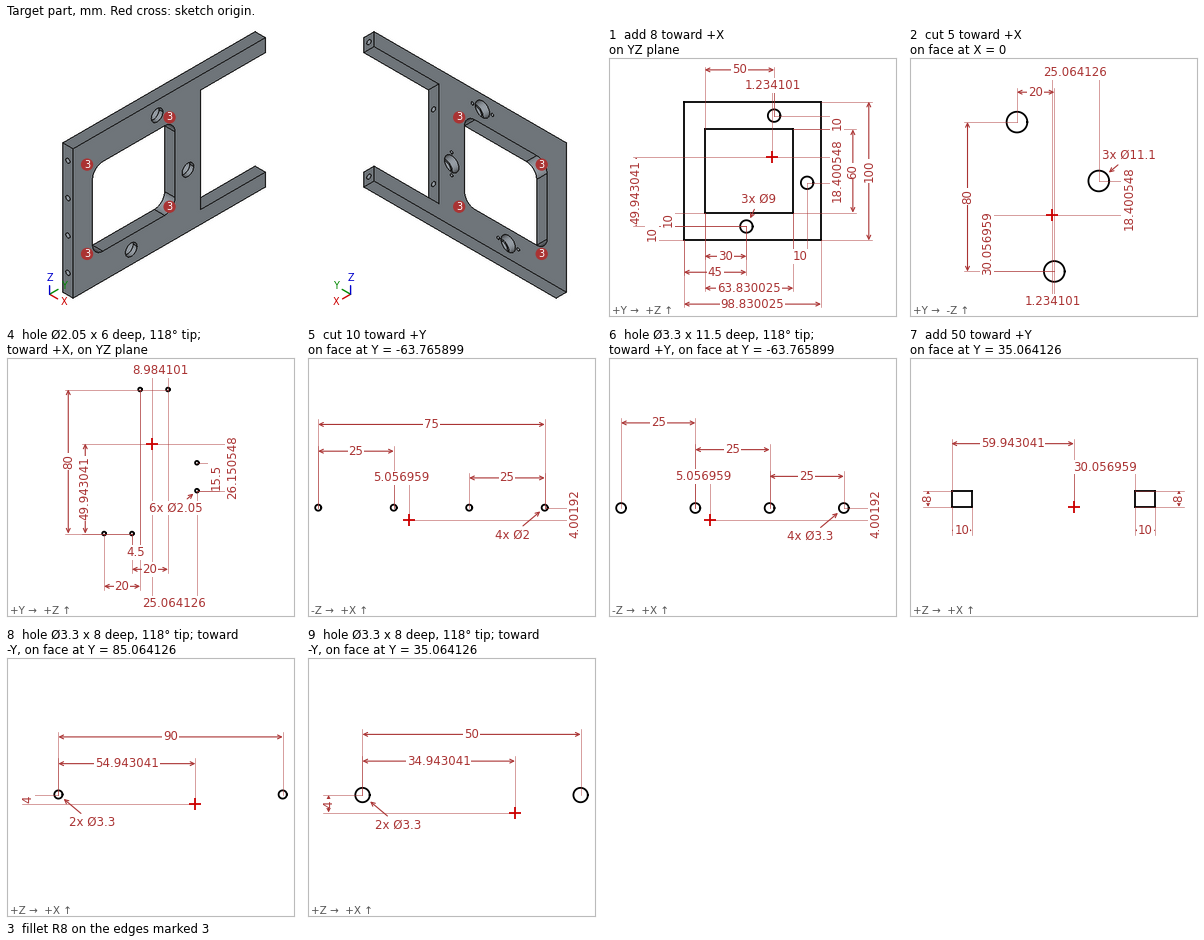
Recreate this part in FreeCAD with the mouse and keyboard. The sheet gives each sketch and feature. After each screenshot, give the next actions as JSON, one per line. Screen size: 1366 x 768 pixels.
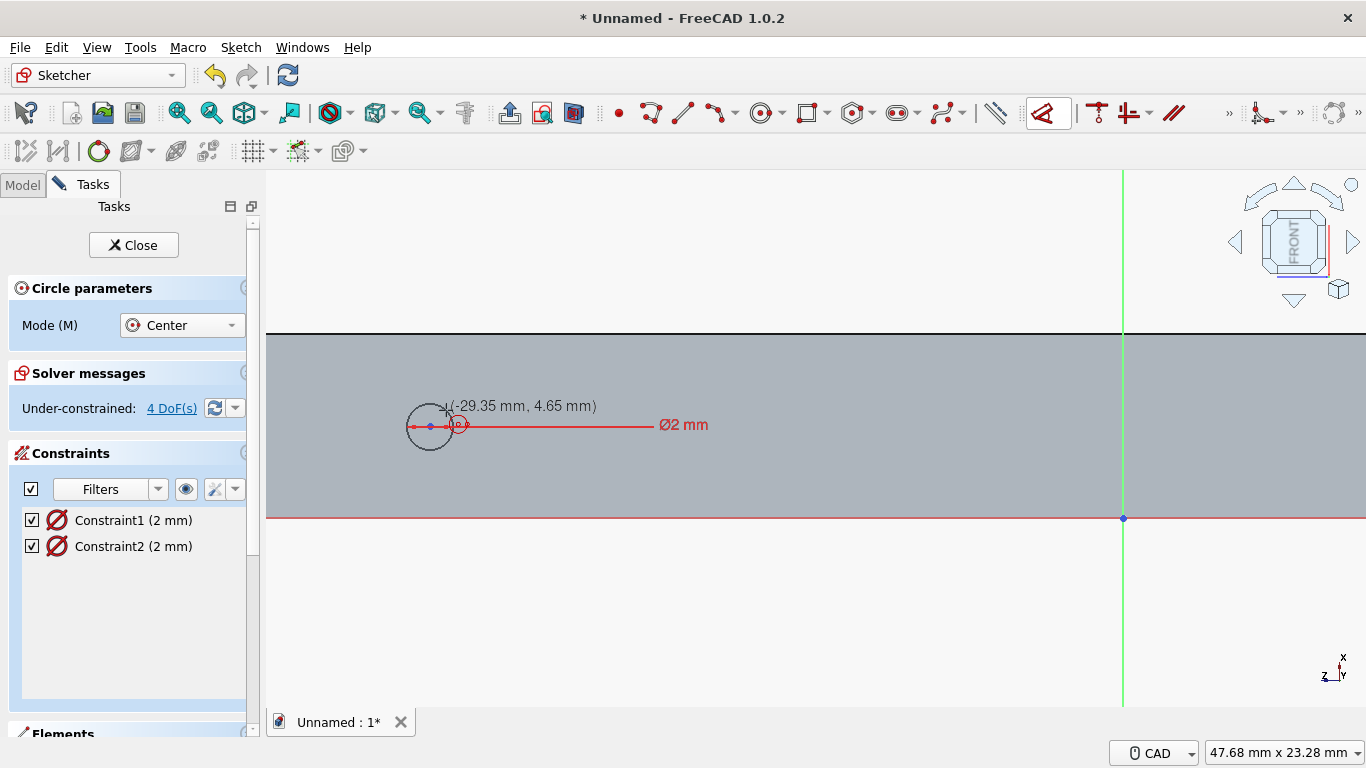
{"action": "scroll", "coordinate": [429, 426], "scroll_direction": "down", "scroll_amount": 5}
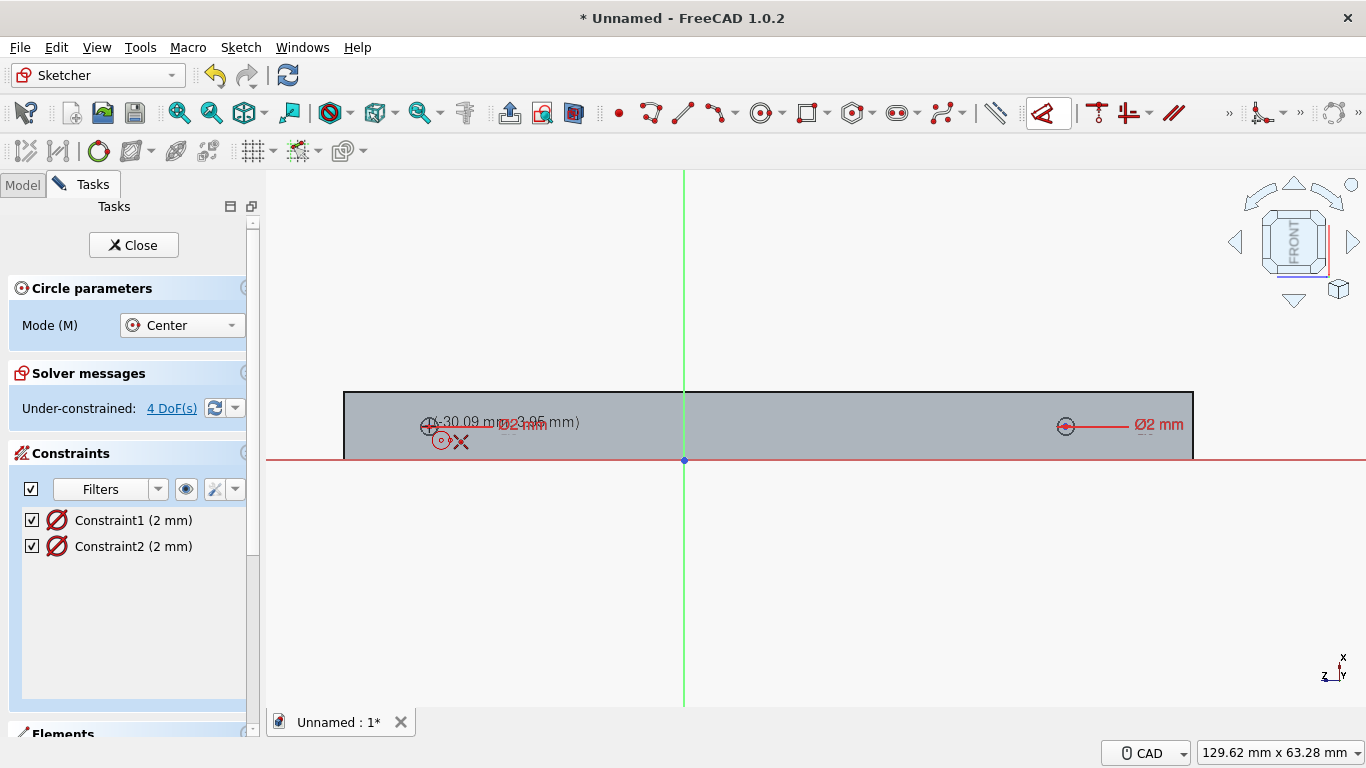
{"action": "scroll", "coordinate": [854, 426], "scroll_direction": "up", "scroll_amount": 5}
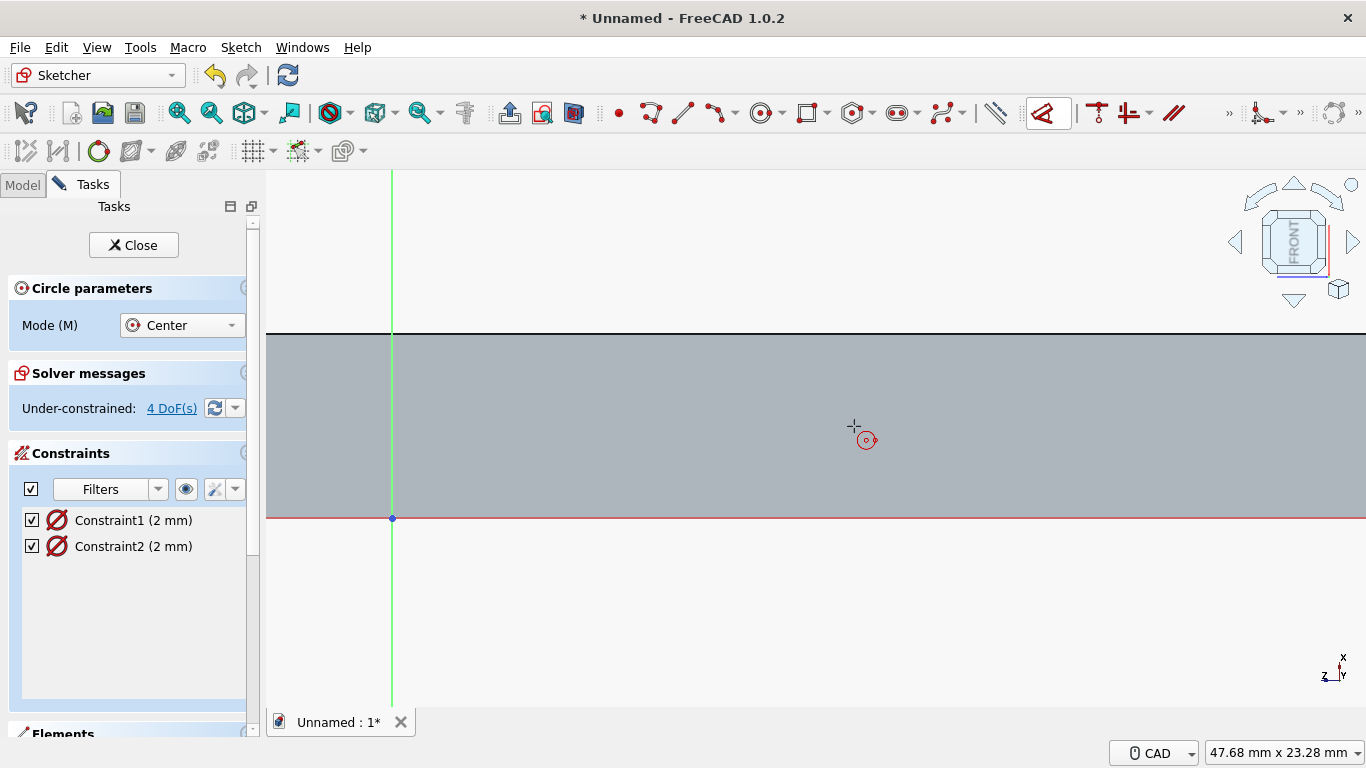
{"action": "left_click", "coordinate": [852, 426]}
{"action": "mouse_move", "coordinate": [869, 410]}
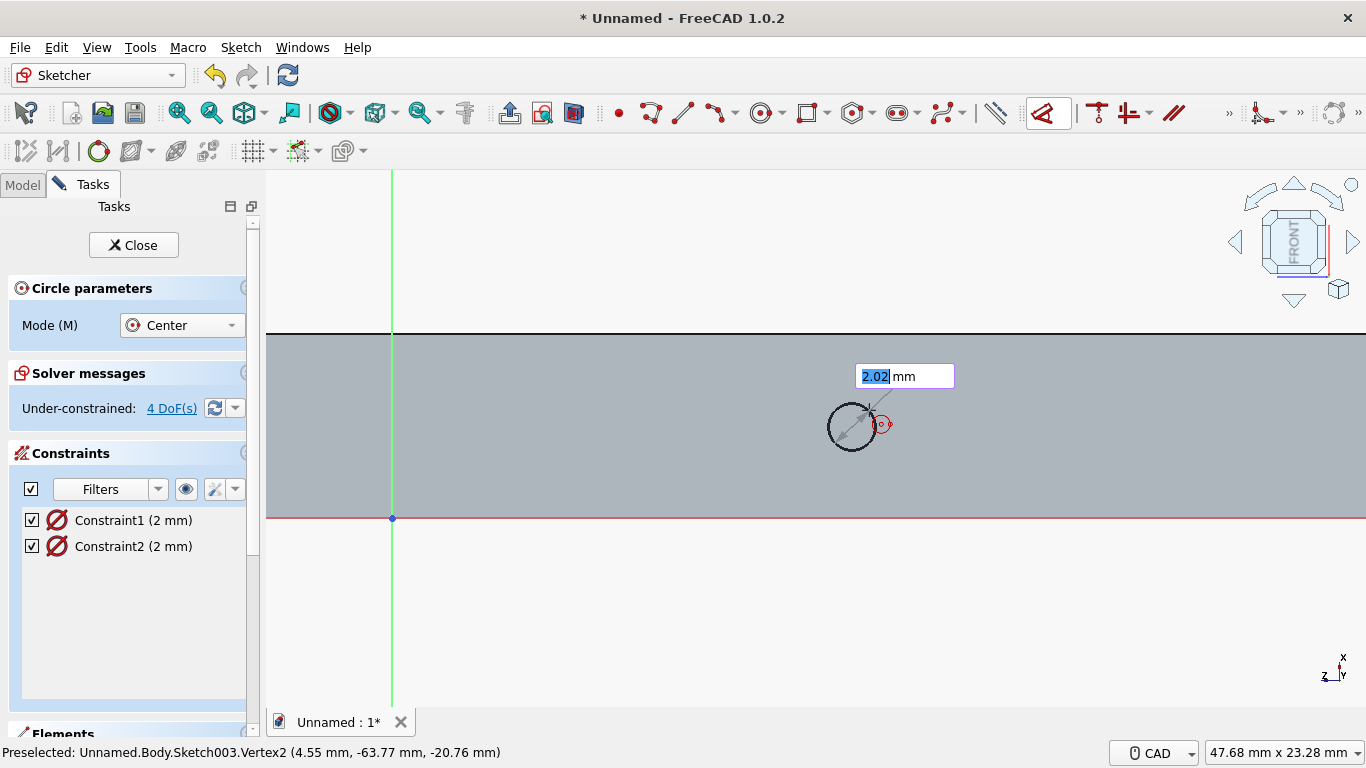
{"action": "type", "text": "2"}
{"action": "key", "text": "Return"}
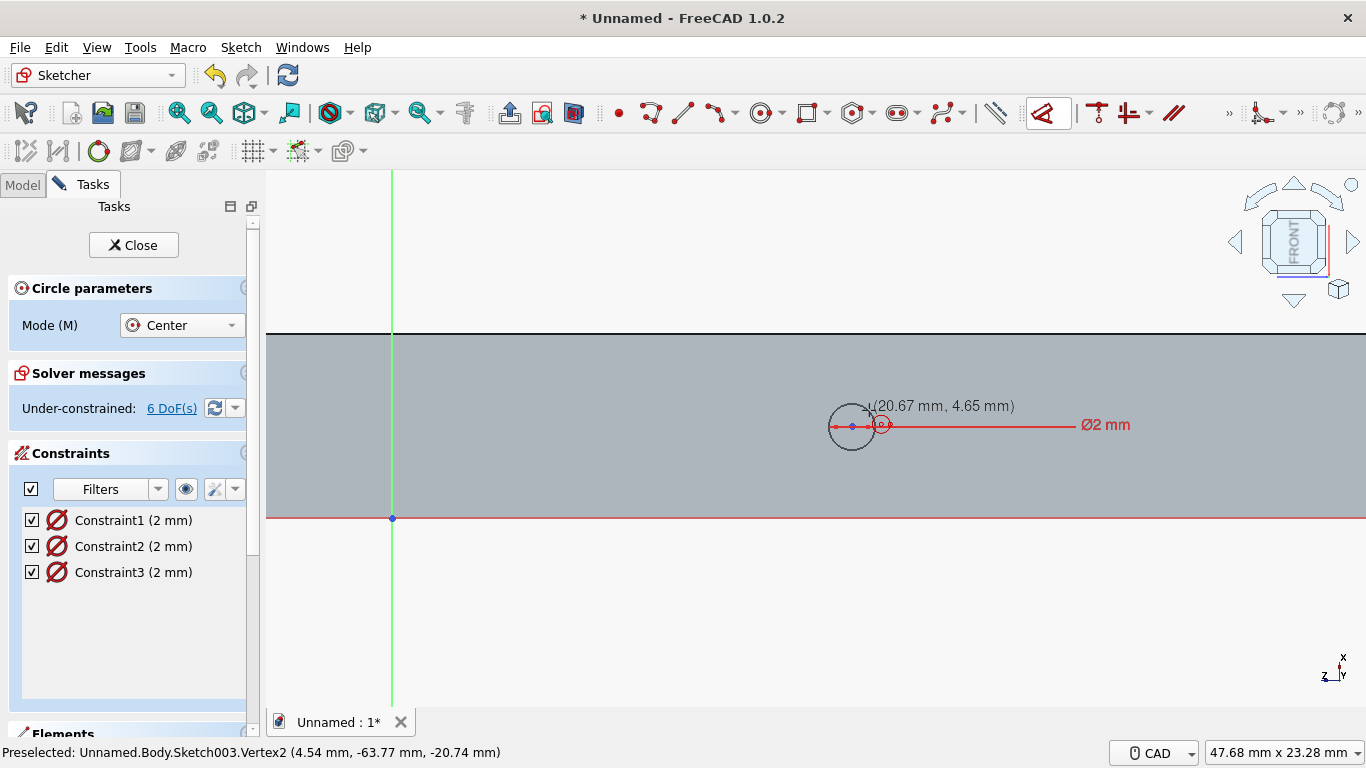
{"action": "scroll", "coordinate": [854, 426], "scroll_direction": "down", "scroll_amount": 5}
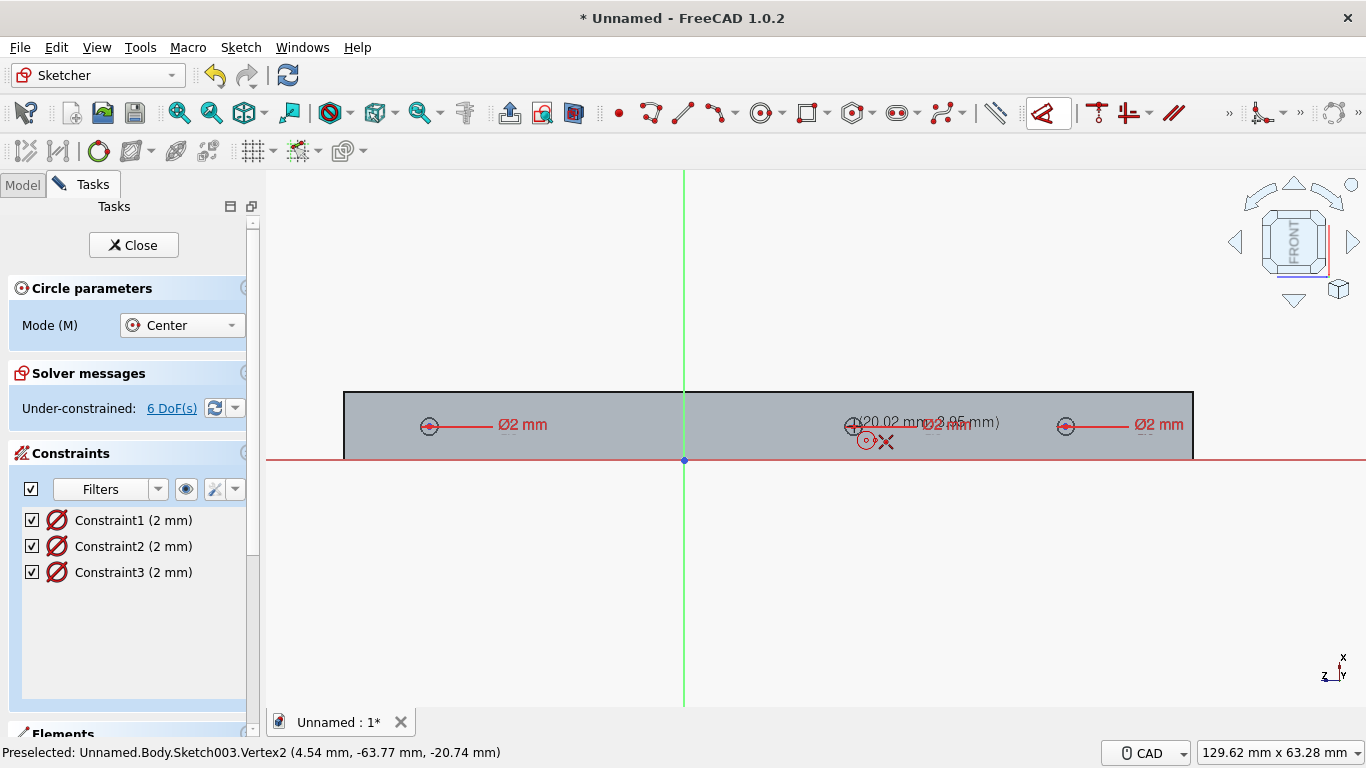
{"action": "scroll", "coordinate": [642, 426], "scroll_direction": "up", "scroll_amount": 5}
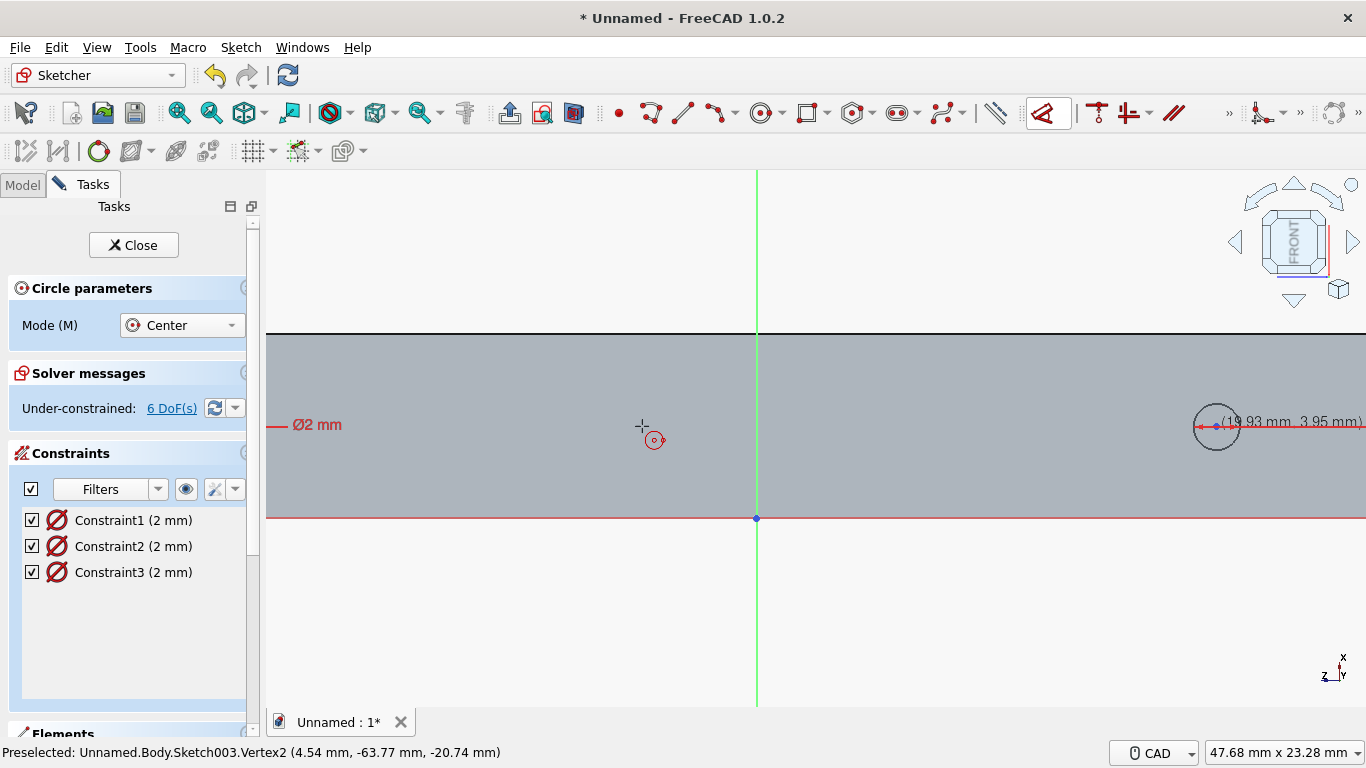
{"action": "left_click", "coordinate": [640, 426]}
{"action": "mouse_move", "coordinate": [656, 410]}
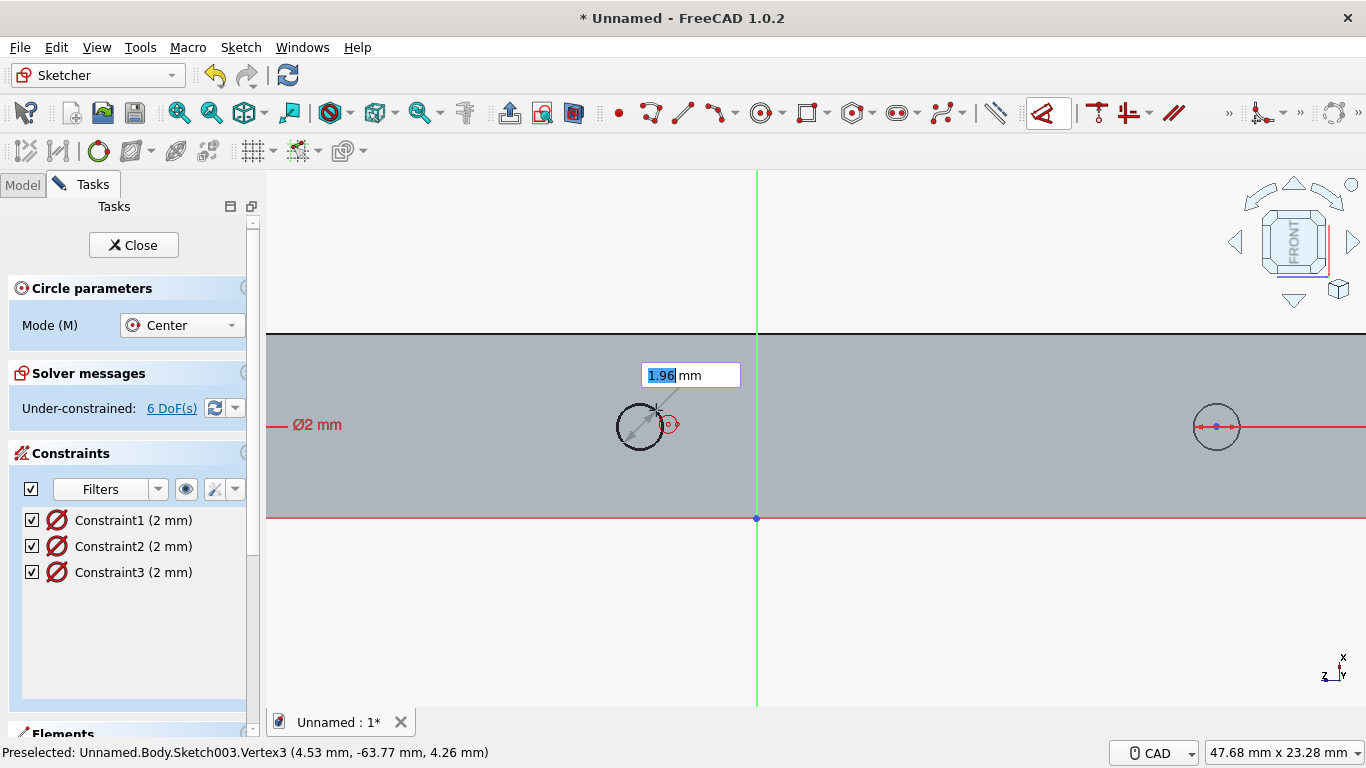
{"action": "type", "text": "2"}
{"action": "key", "text": "Return"}
{"action": "key", "text": "Escape"}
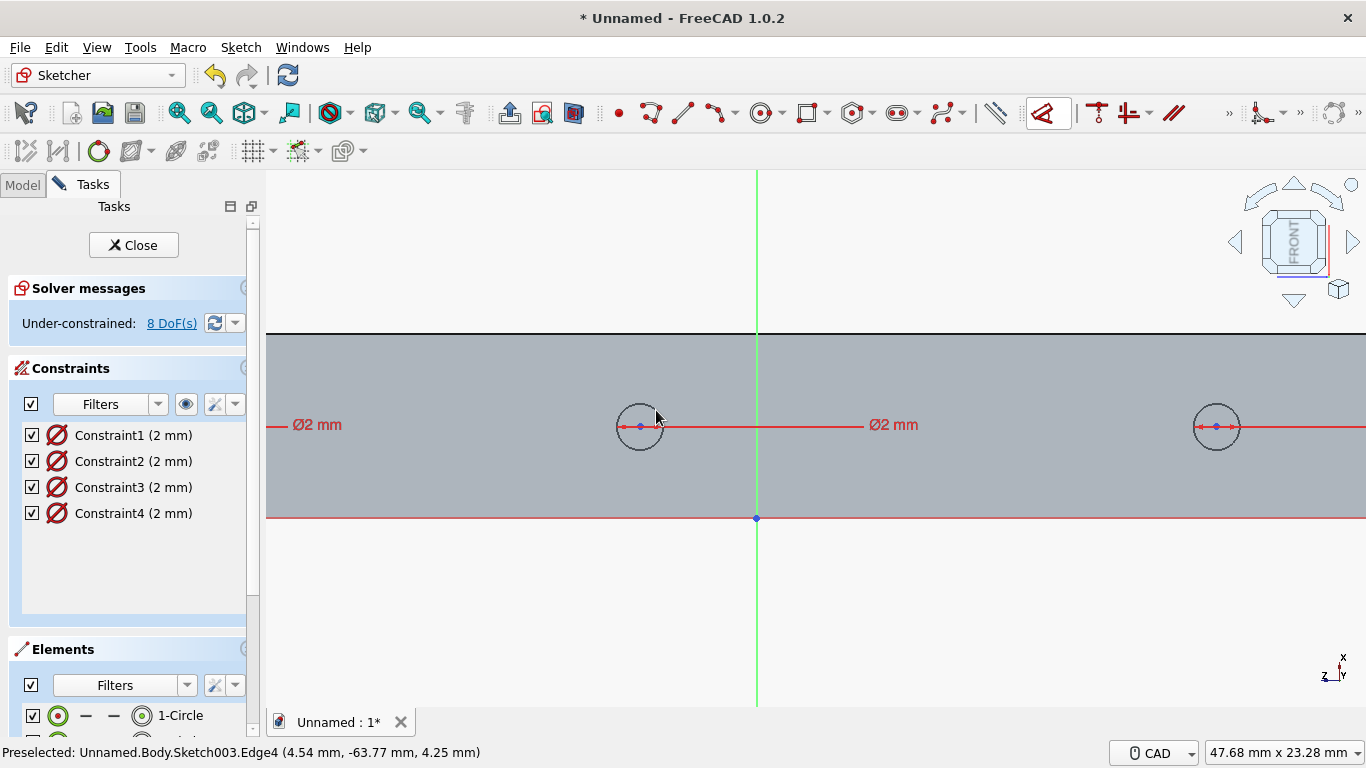
{"action": "scroll", "coordinate": [642, 426], "scroll_direction": "down", "scroll_amount": 5}